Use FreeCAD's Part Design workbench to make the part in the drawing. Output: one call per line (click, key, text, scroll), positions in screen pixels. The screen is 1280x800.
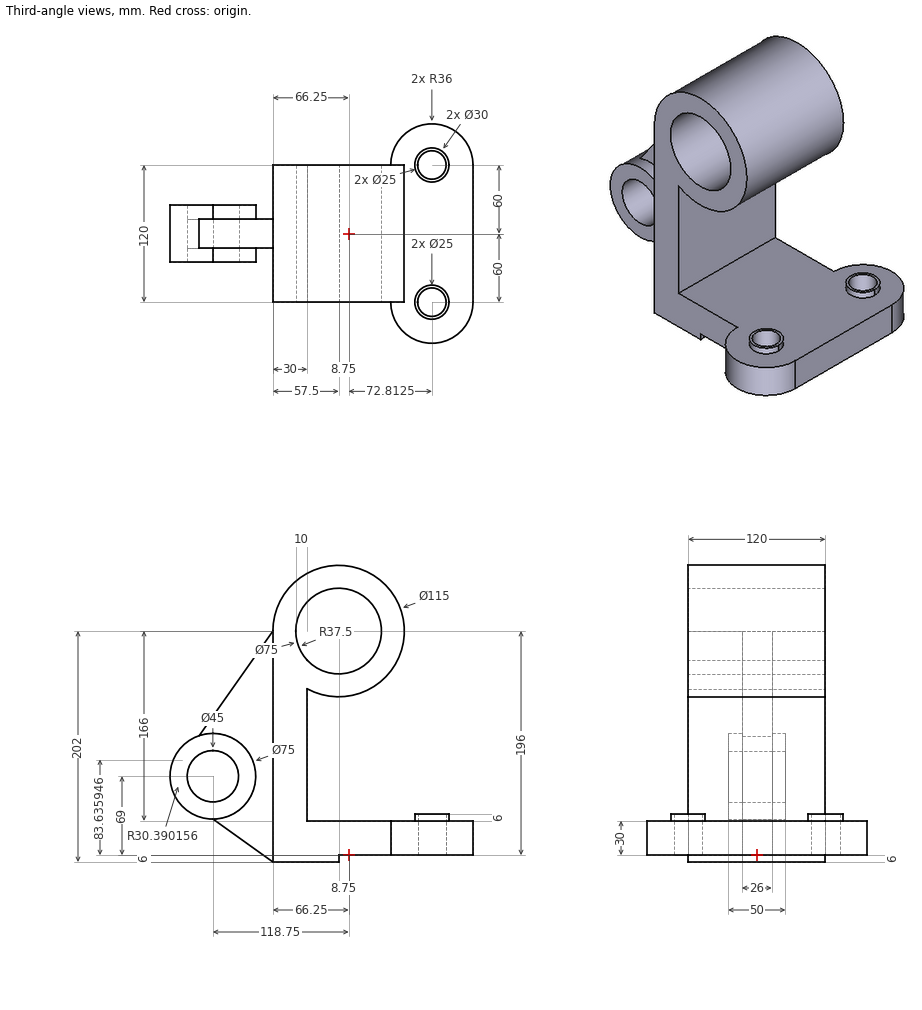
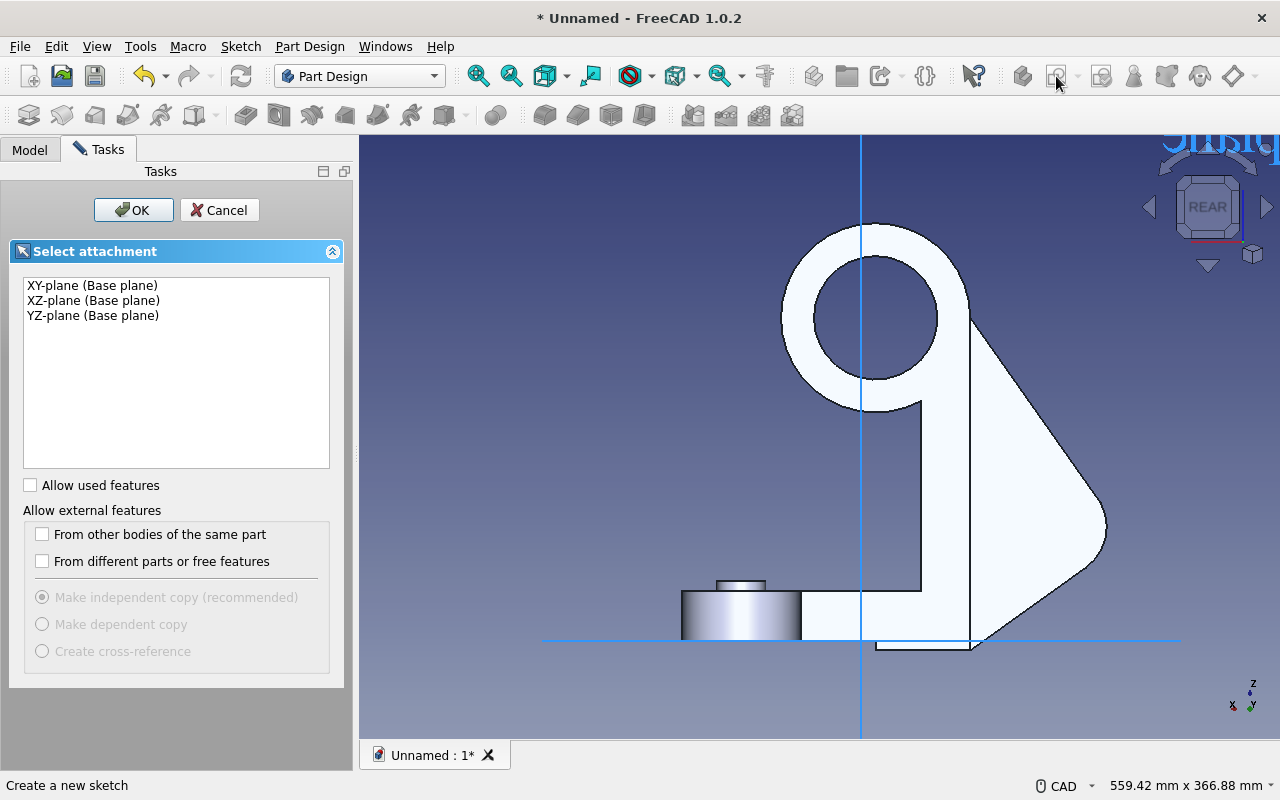
click(84, 300)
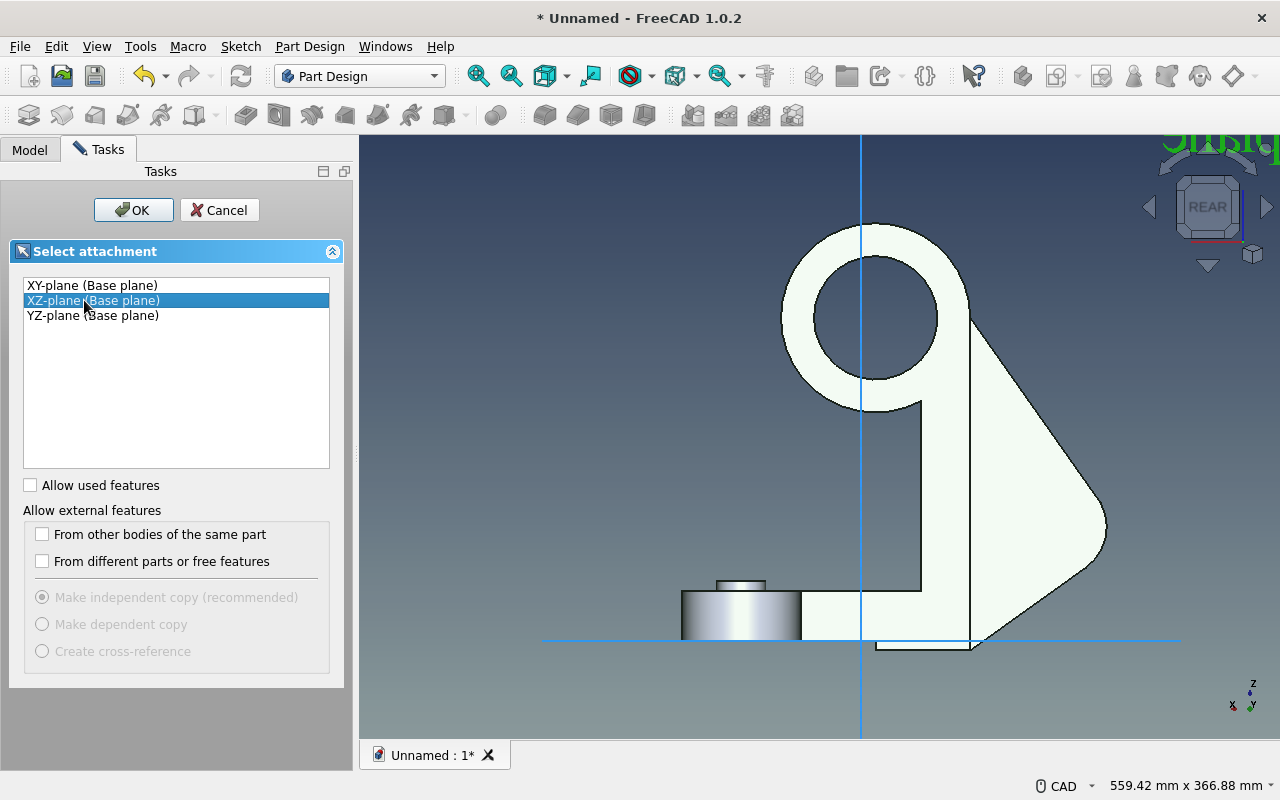
click(134, 210)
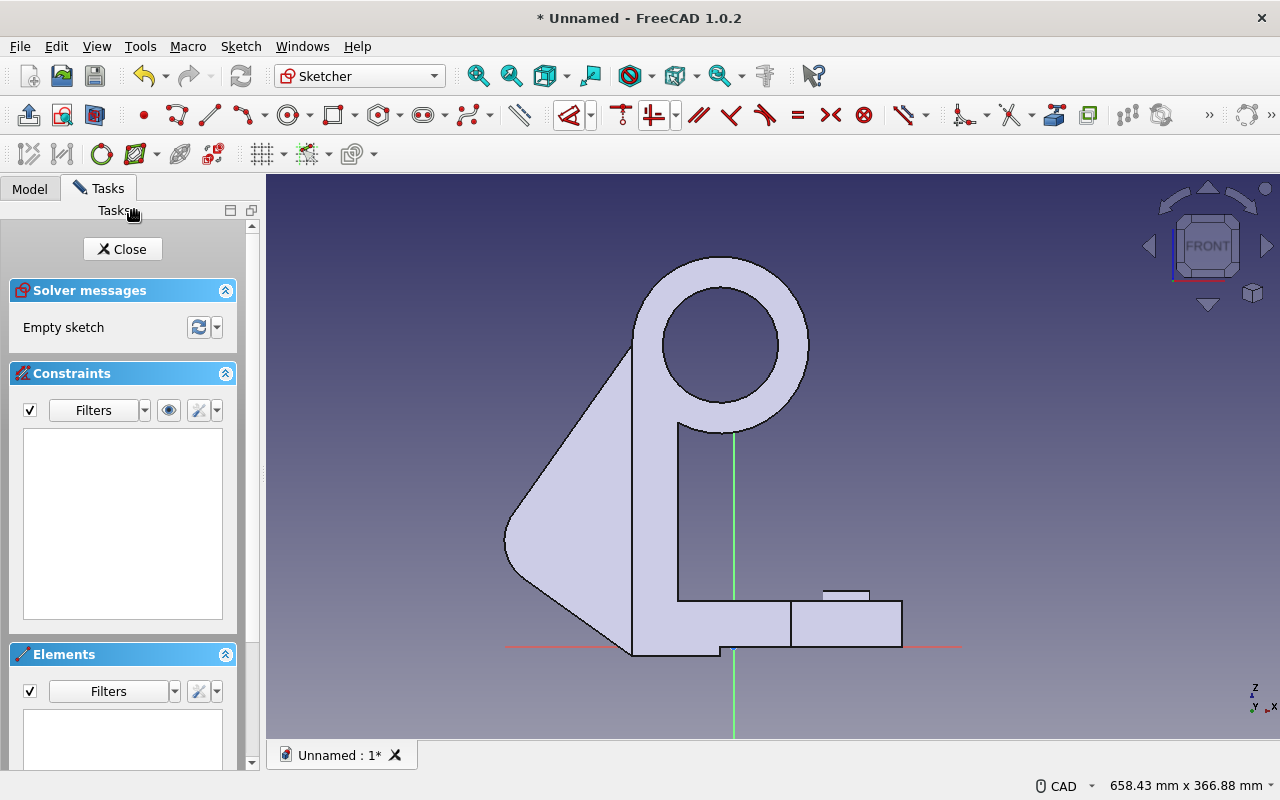
click(95, 116)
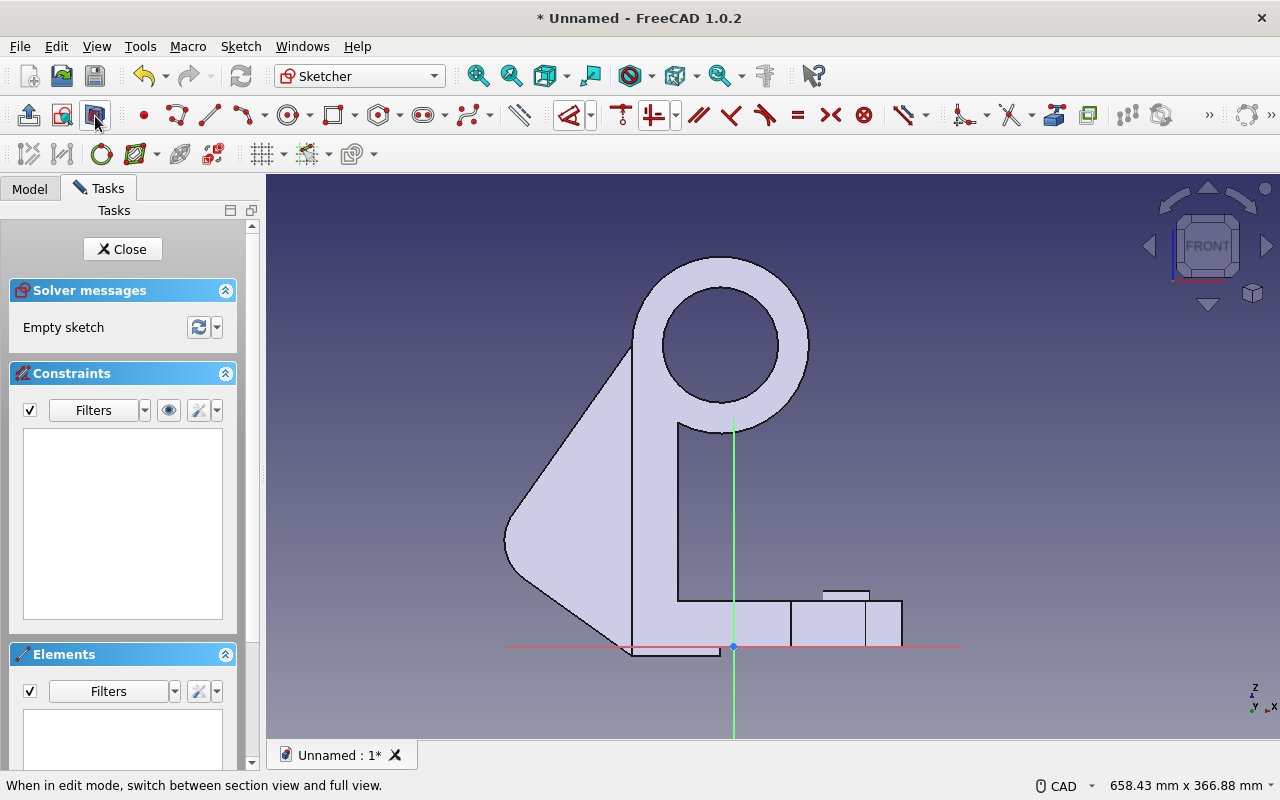
scroll(540, 653, up, 4)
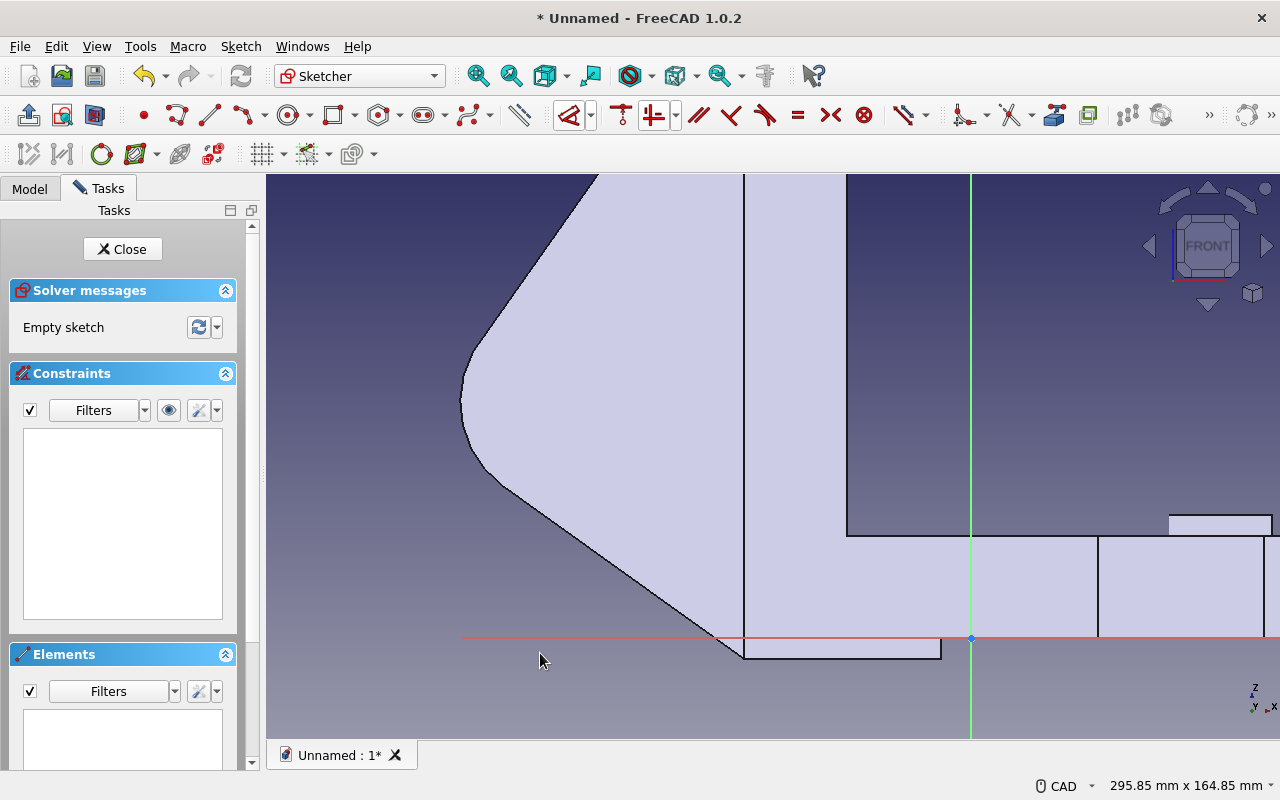
key(g)
key(c)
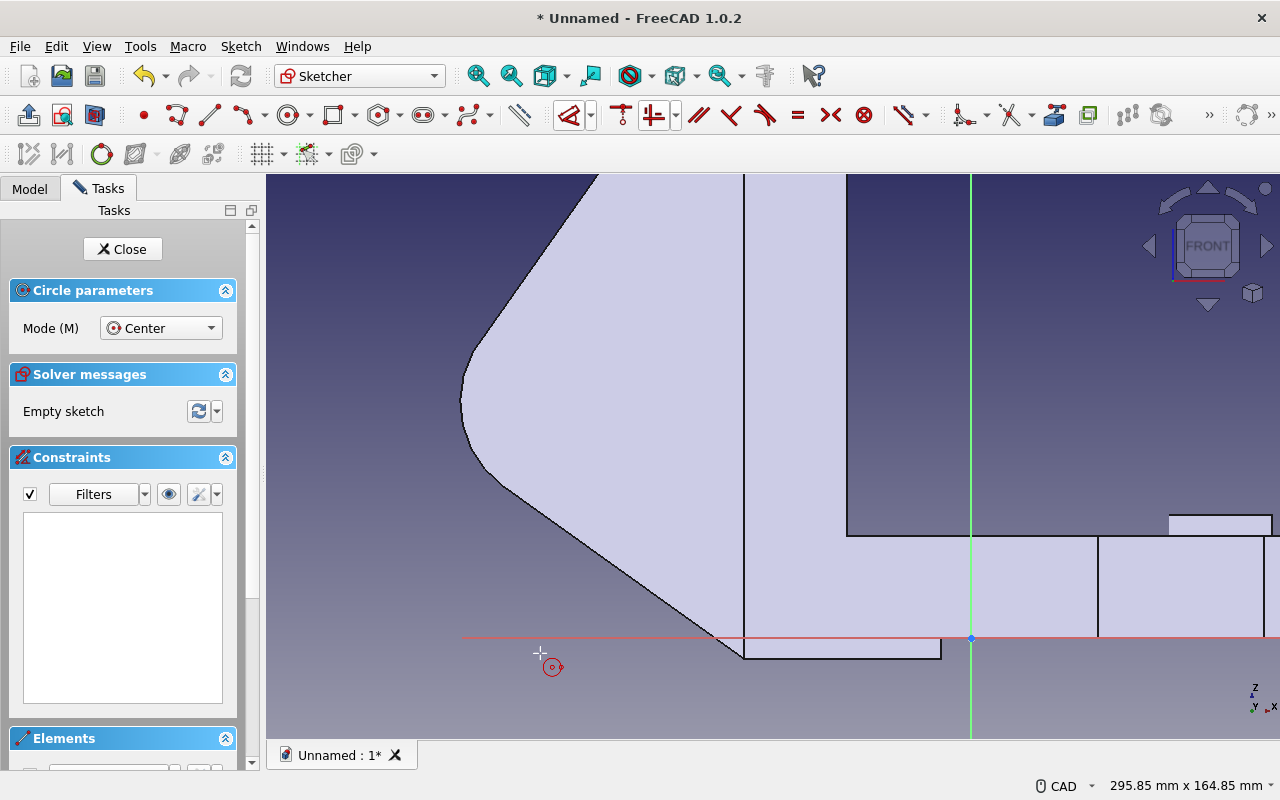
click(564, 402)
click(655, 311)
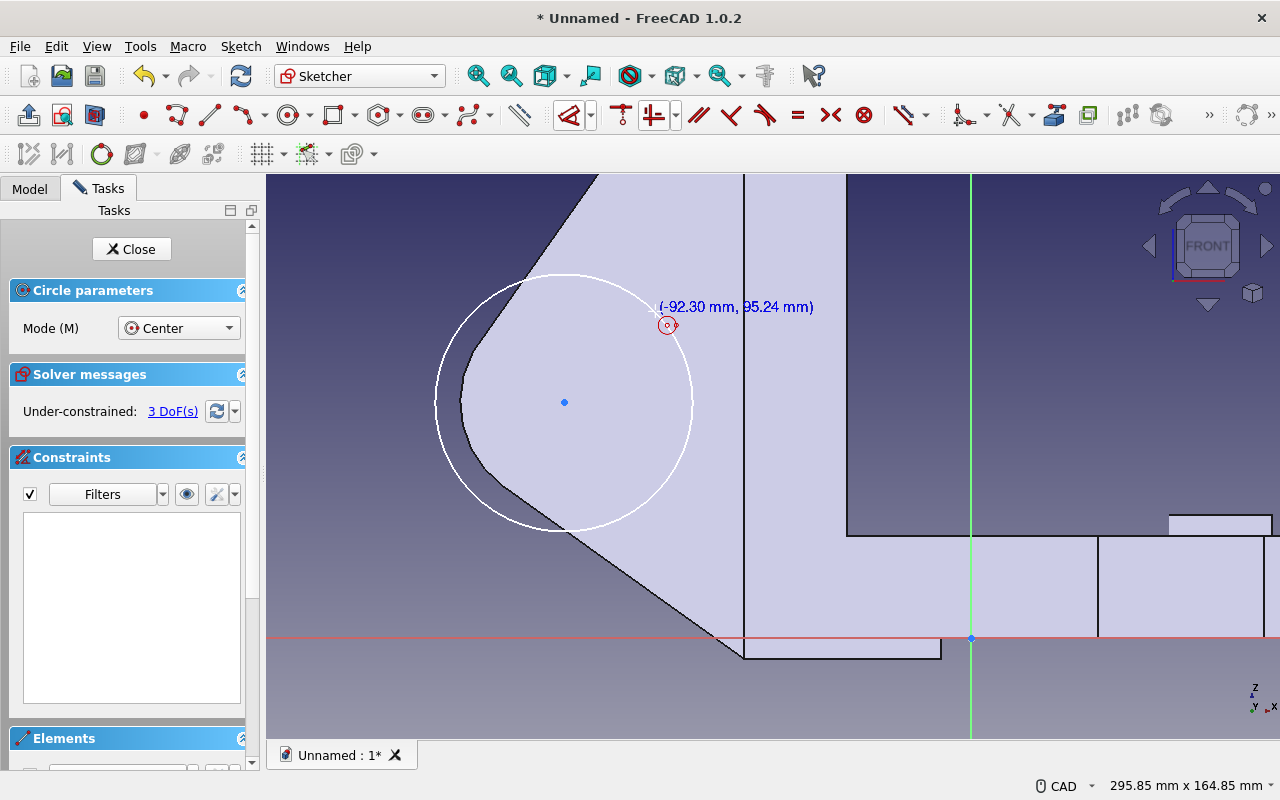
click(564, 403)
click(619, 347)
key(Escape)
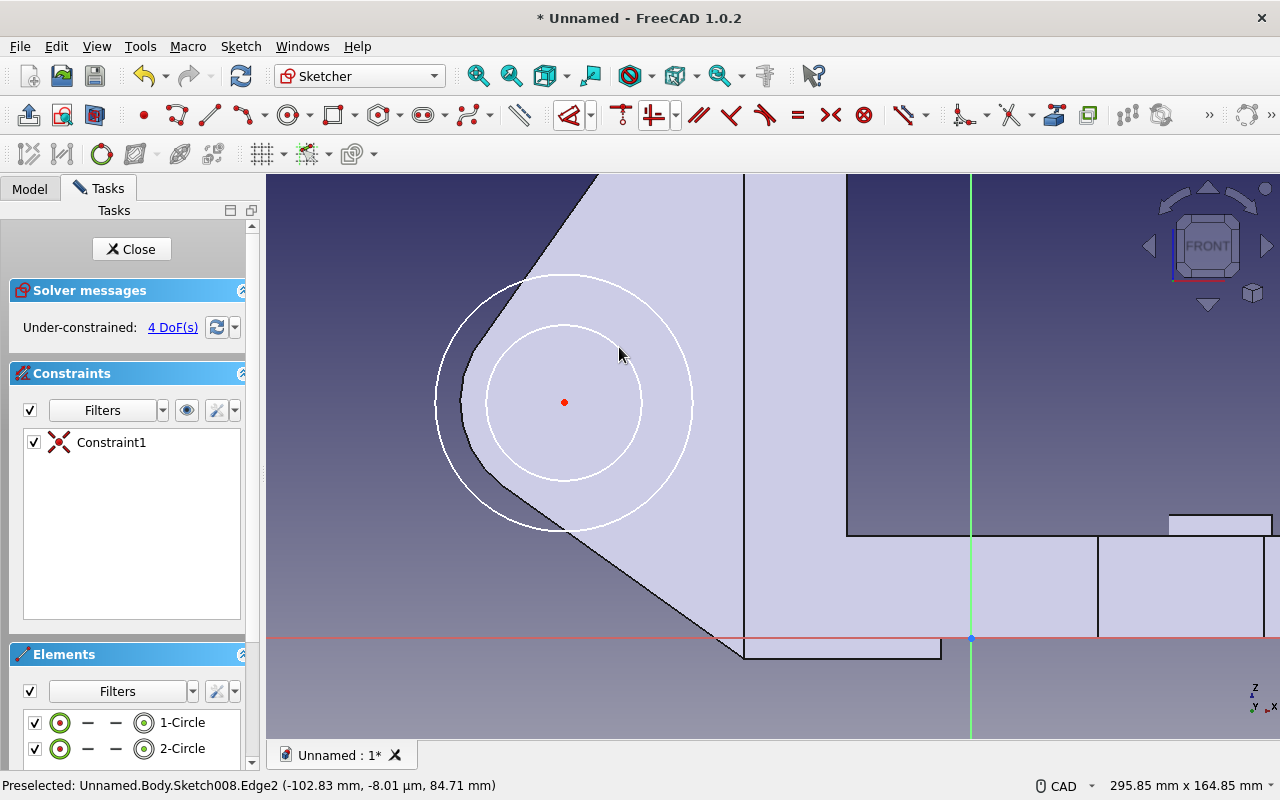
click(655, 312)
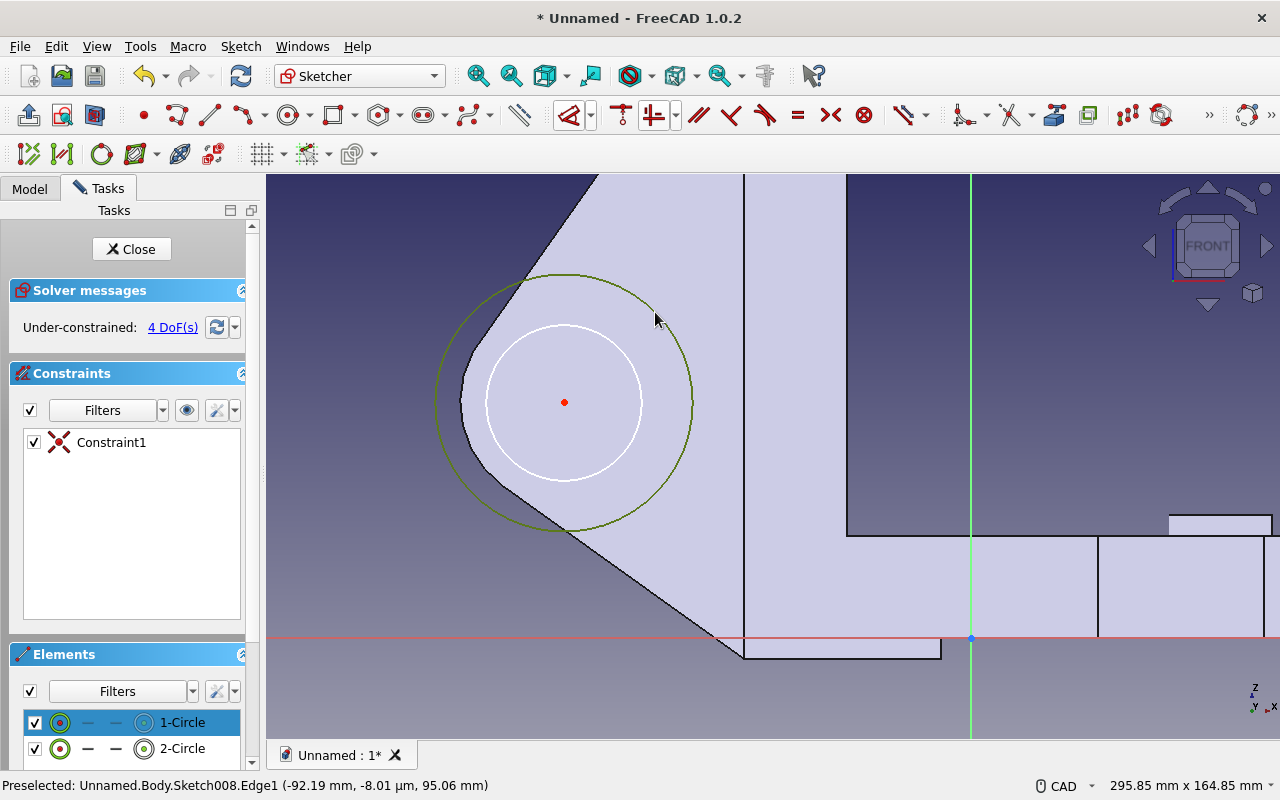
key(k)
key(o)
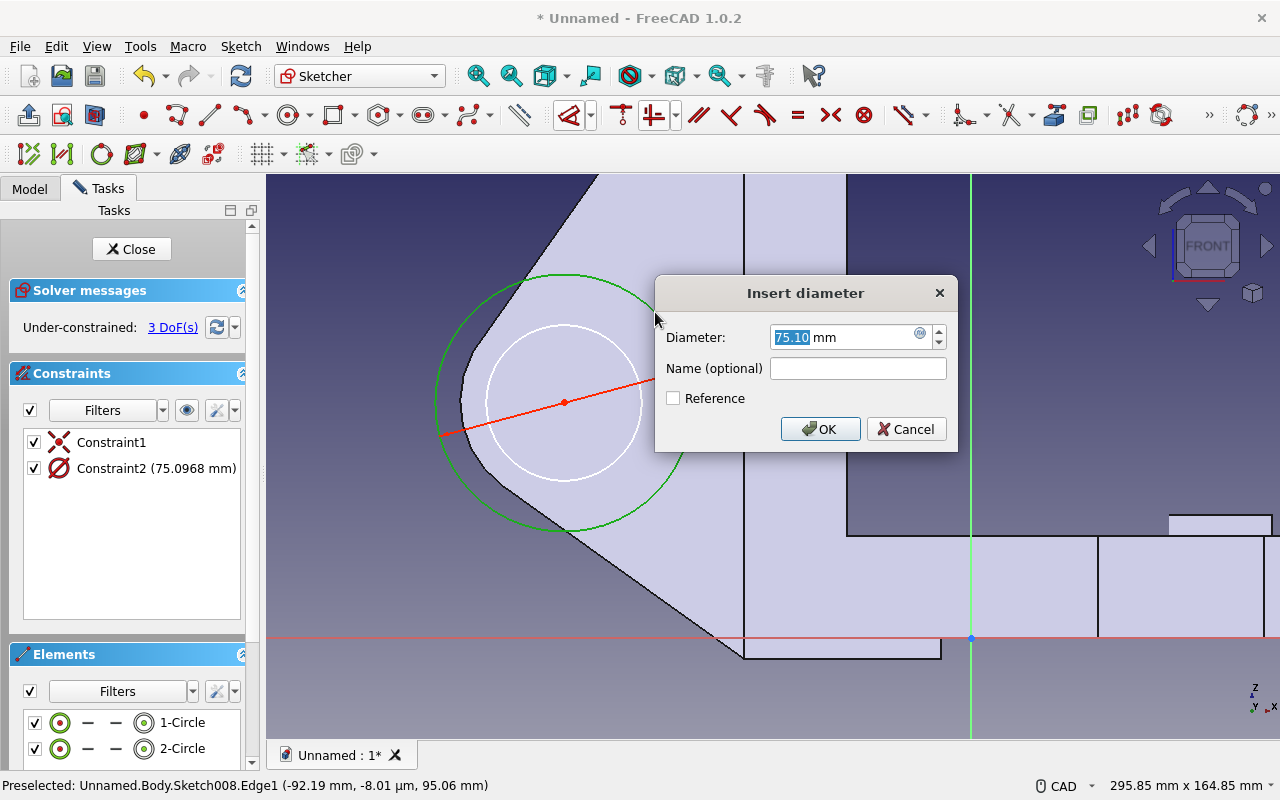
text(75)
key(Return)